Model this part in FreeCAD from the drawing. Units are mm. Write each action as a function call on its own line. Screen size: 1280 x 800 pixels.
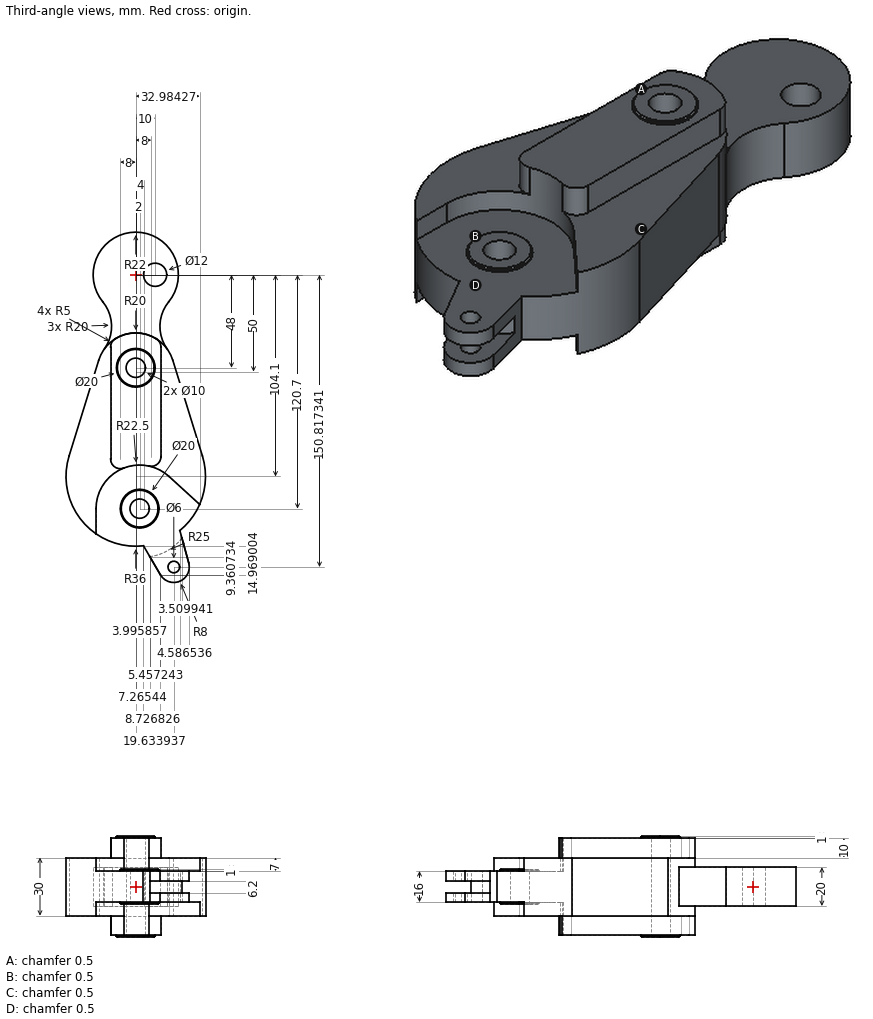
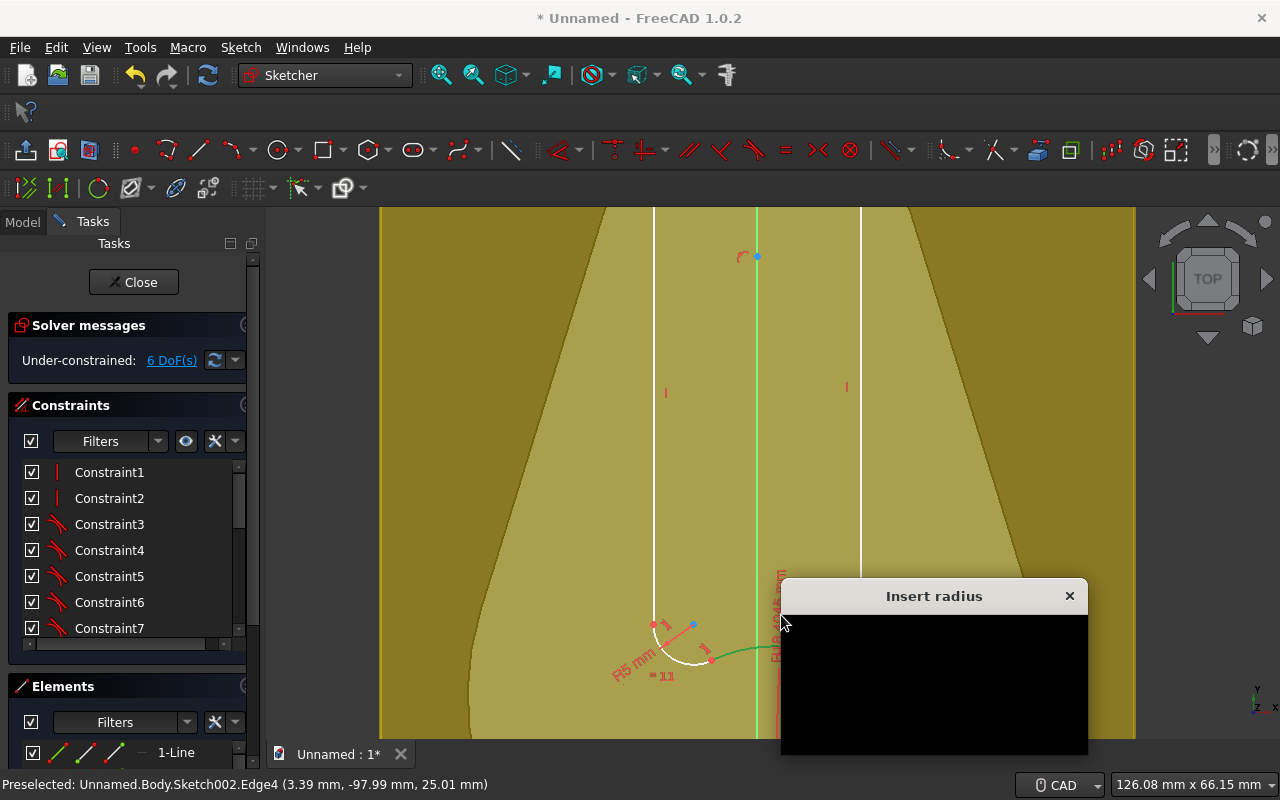
text(22.5)
key(Return)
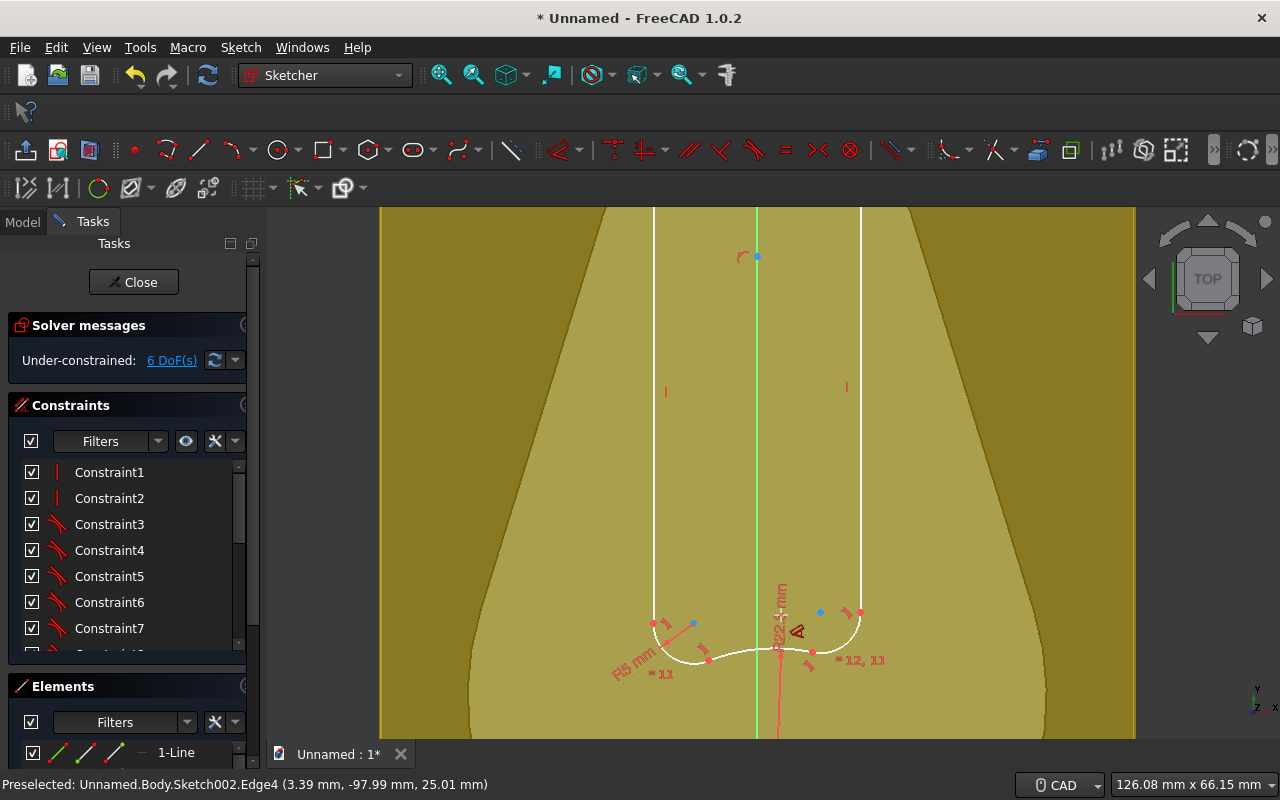
scroll(662, 647, down, 4)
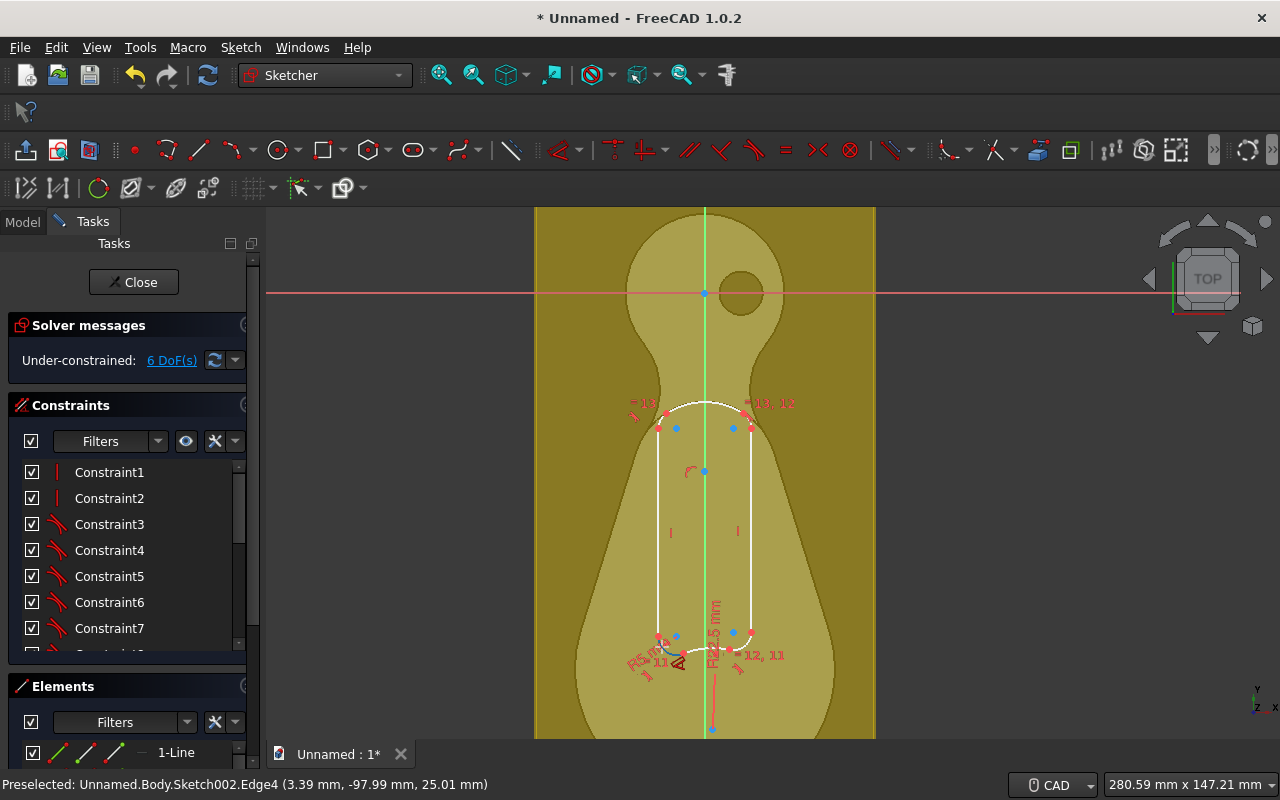
click(721, 404)
click(728, 373)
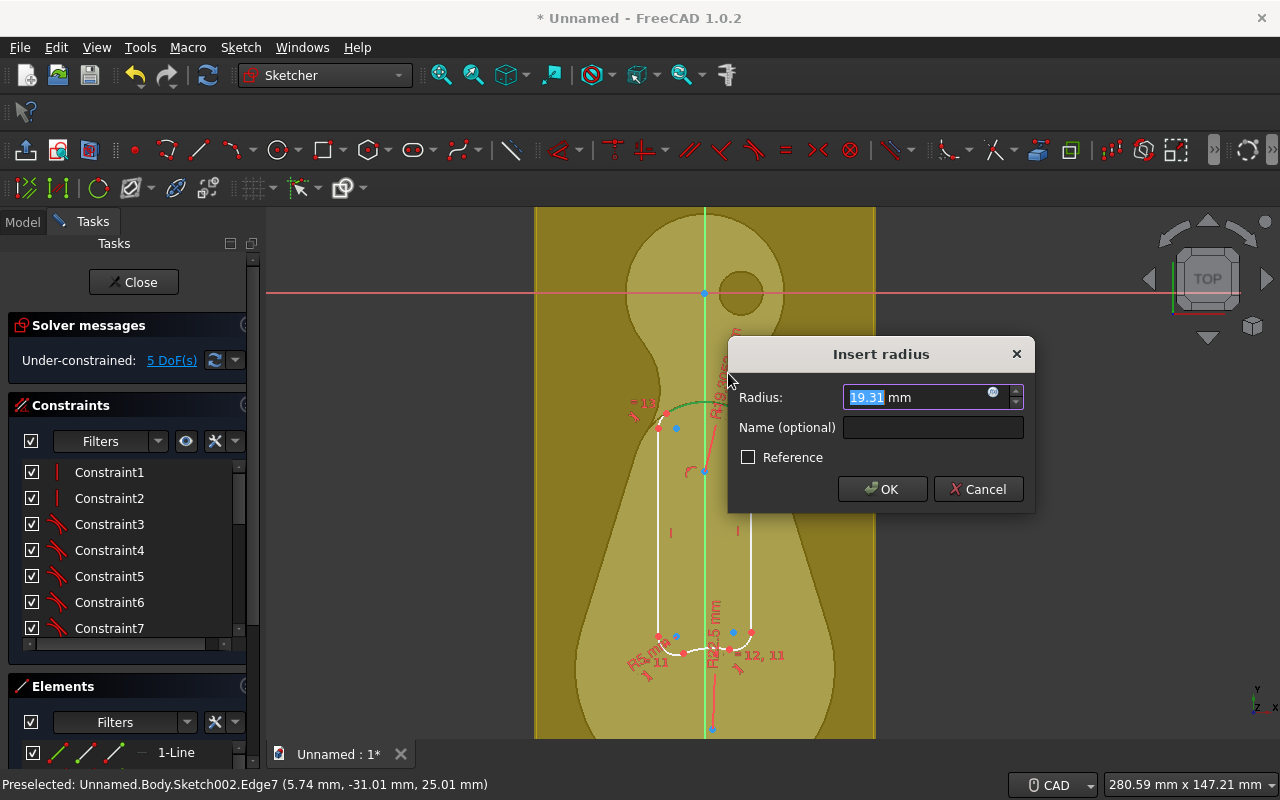
text(20)
key(Return)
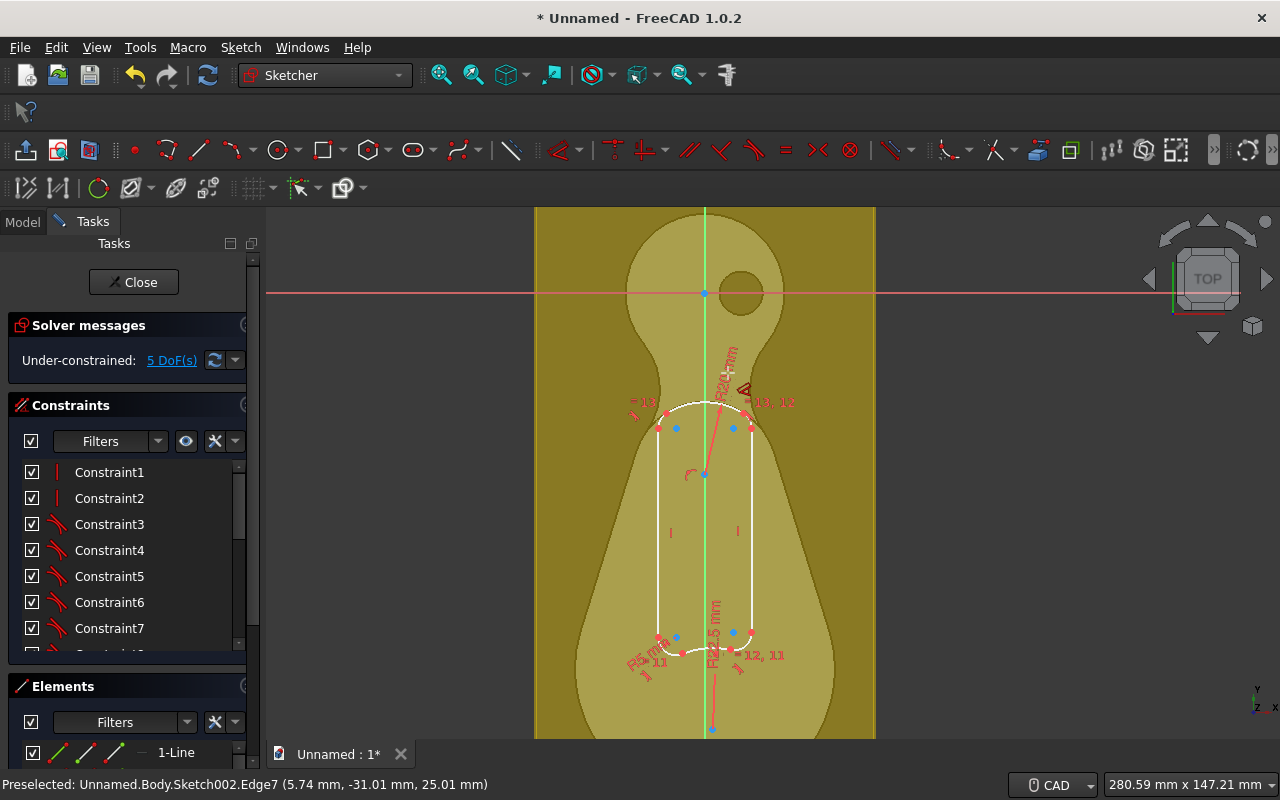
scroll(676, 637, up, 2)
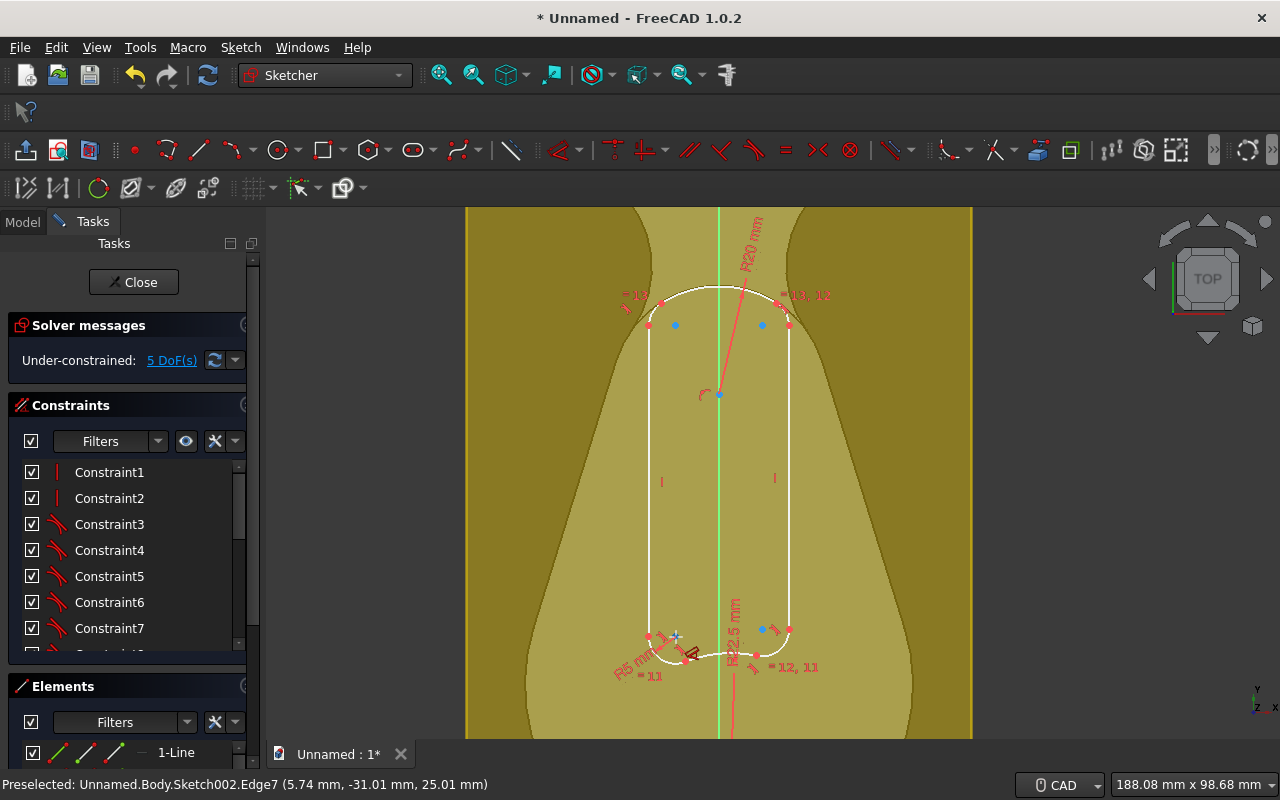
click(676, 637)
click(697, 695)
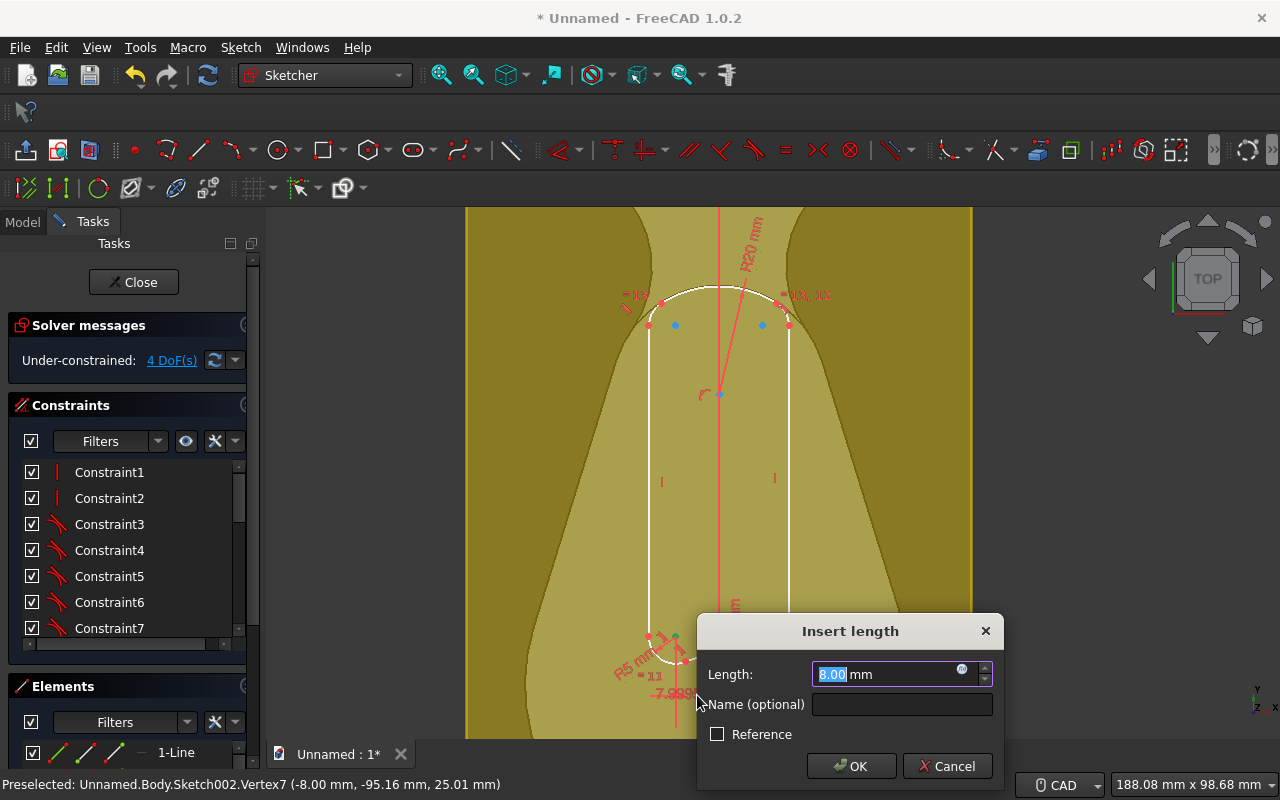
text(8)
key(Return)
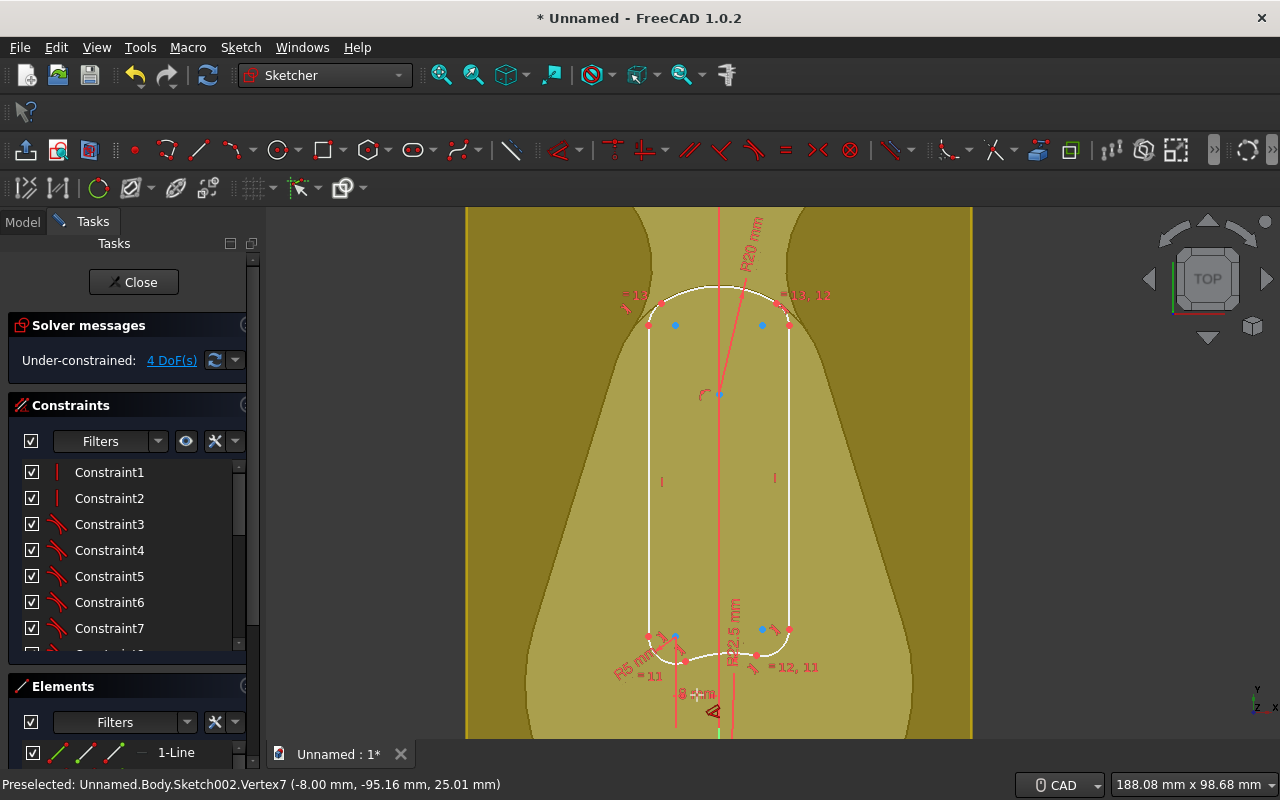
scroll(675, 636, down, 2)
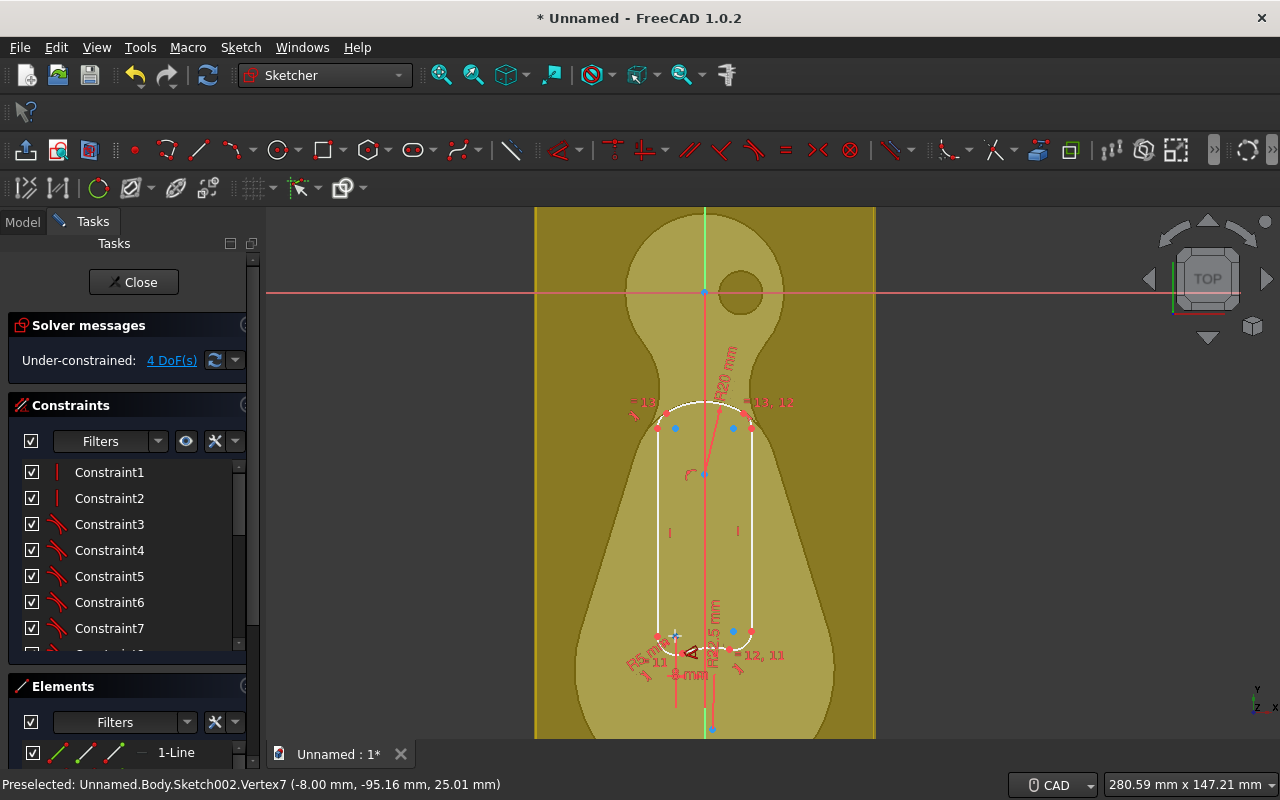
scroll(704, 301, down, 1)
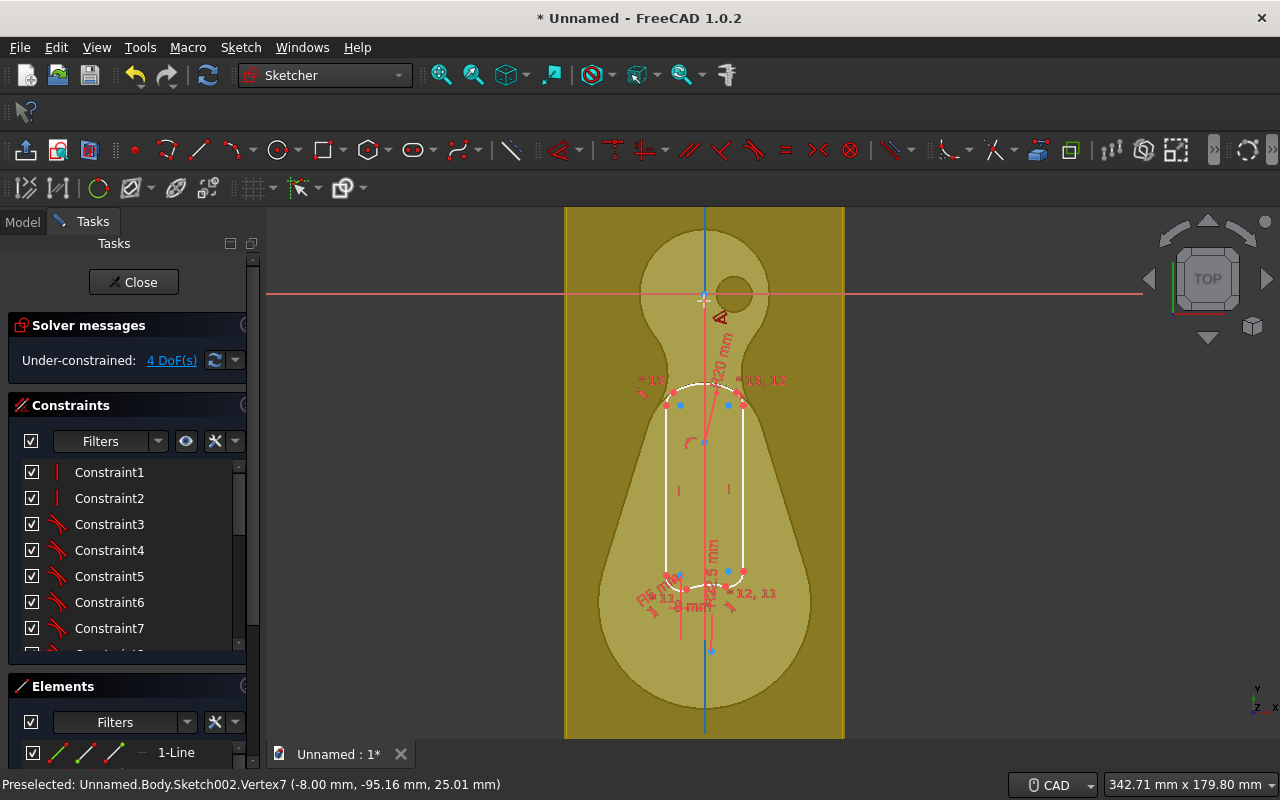
scroll(711, 652, up, 10)